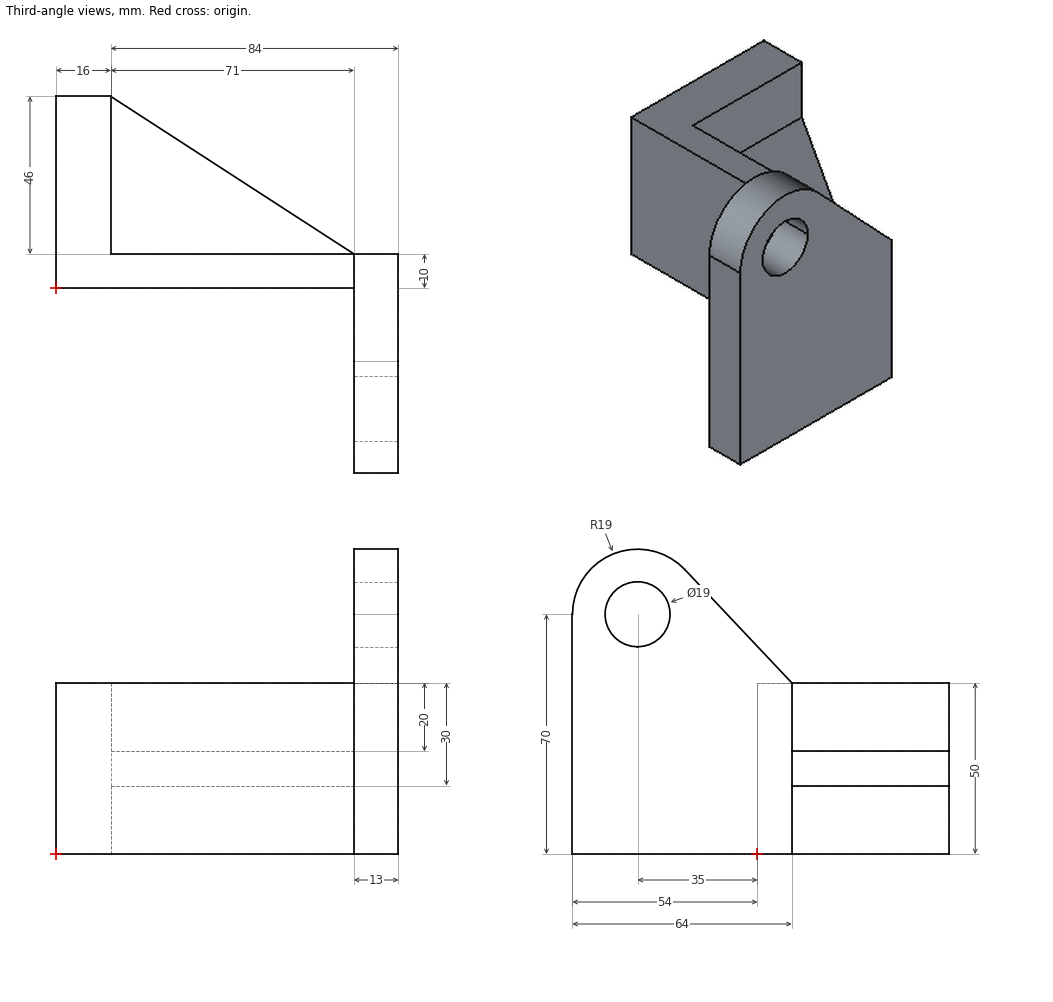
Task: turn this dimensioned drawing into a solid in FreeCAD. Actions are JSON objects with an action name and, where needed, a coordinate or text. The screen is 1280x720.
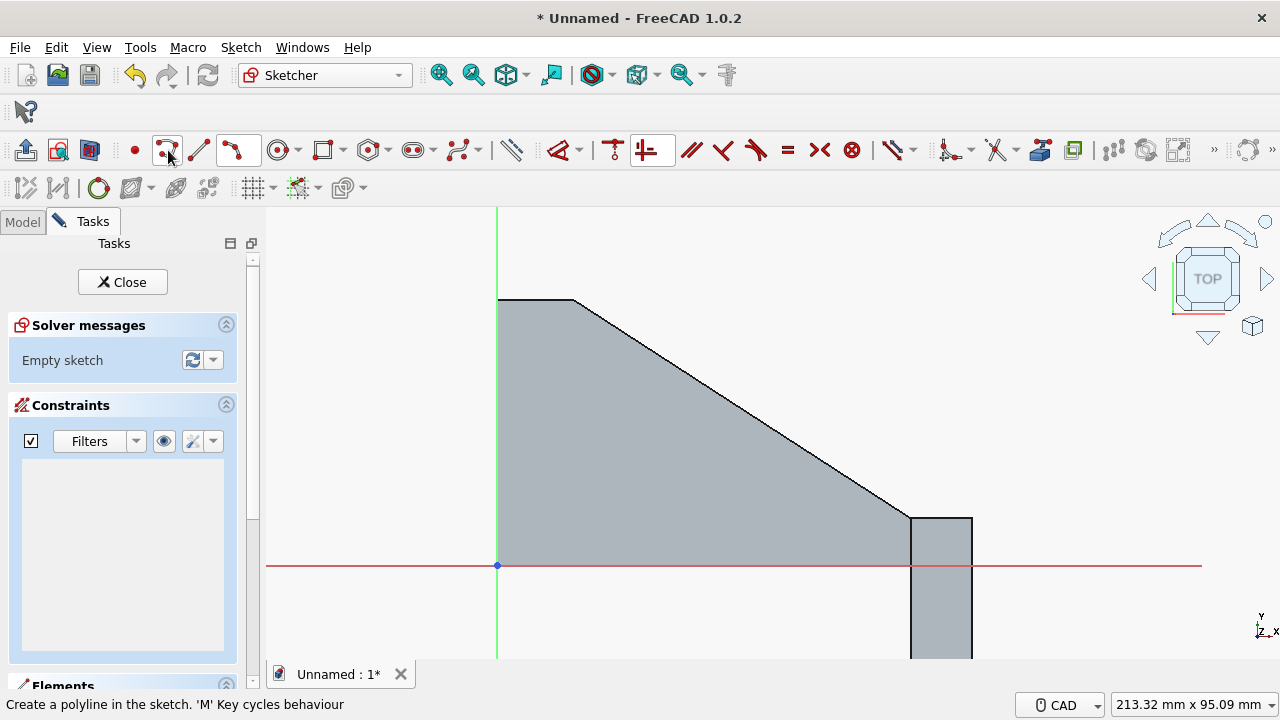
{"action": "left_click", "coordinate": [573, 518]}
{"action": "left_click", "coordinate": [911, 518]}
{"action": "left_click", "coordinate": [573, 300]}
{"action": "left_click", "coordinate": [573, 519]}
{"action": "key", "text": "Escape"}
{"action": "key", "text": "Escape"}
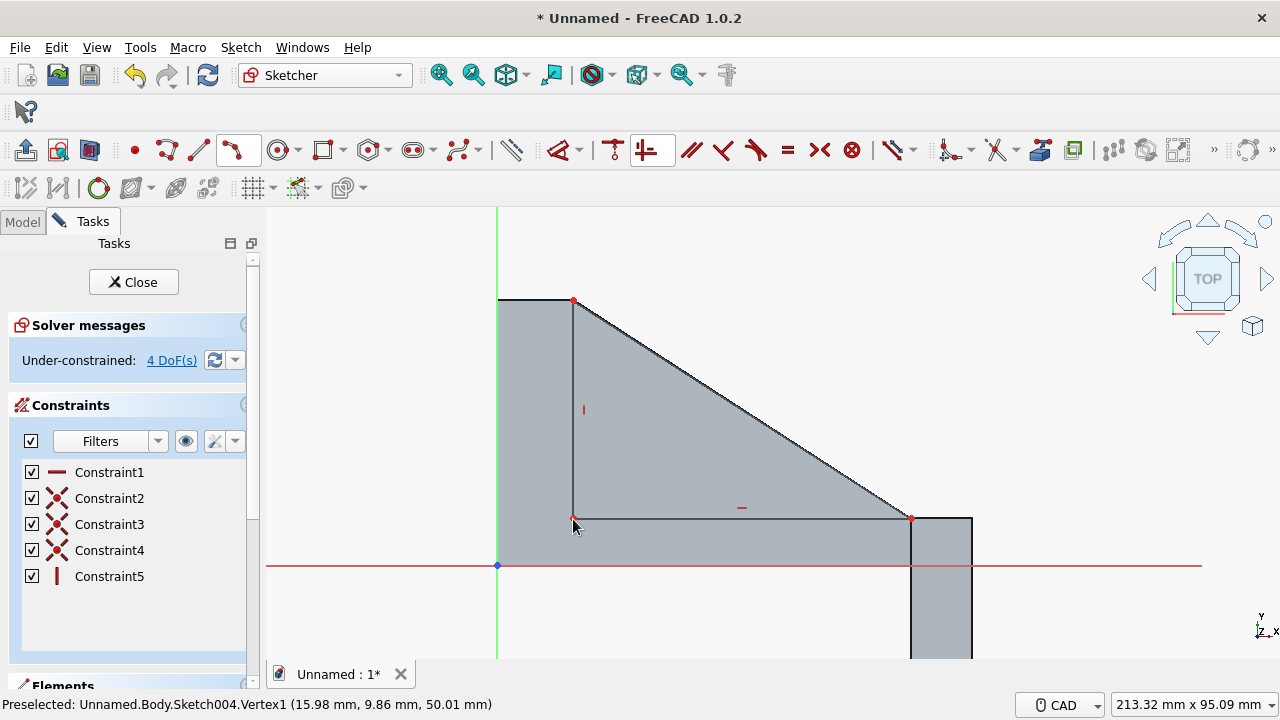
{"action": "key", "text": "d"}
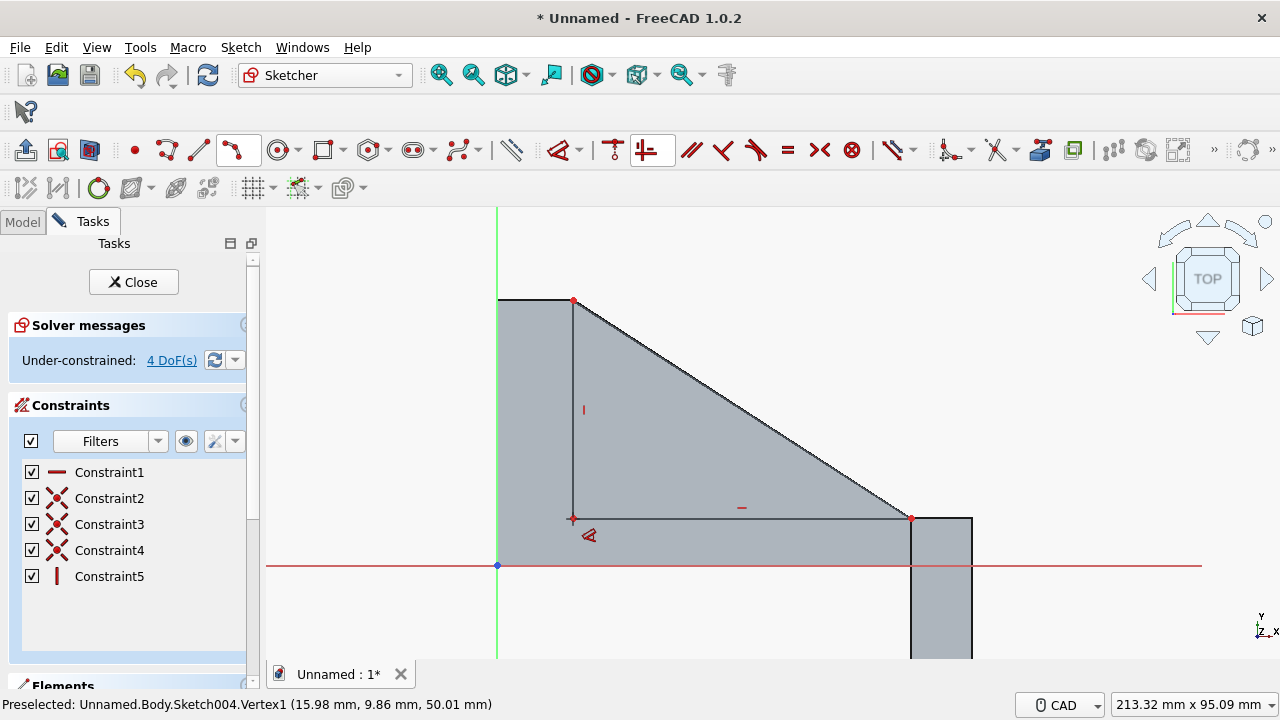
{"action": "left_click", "coordinate": [674, 519]}
{"action": "left_click", "coordinate": [742, 485]}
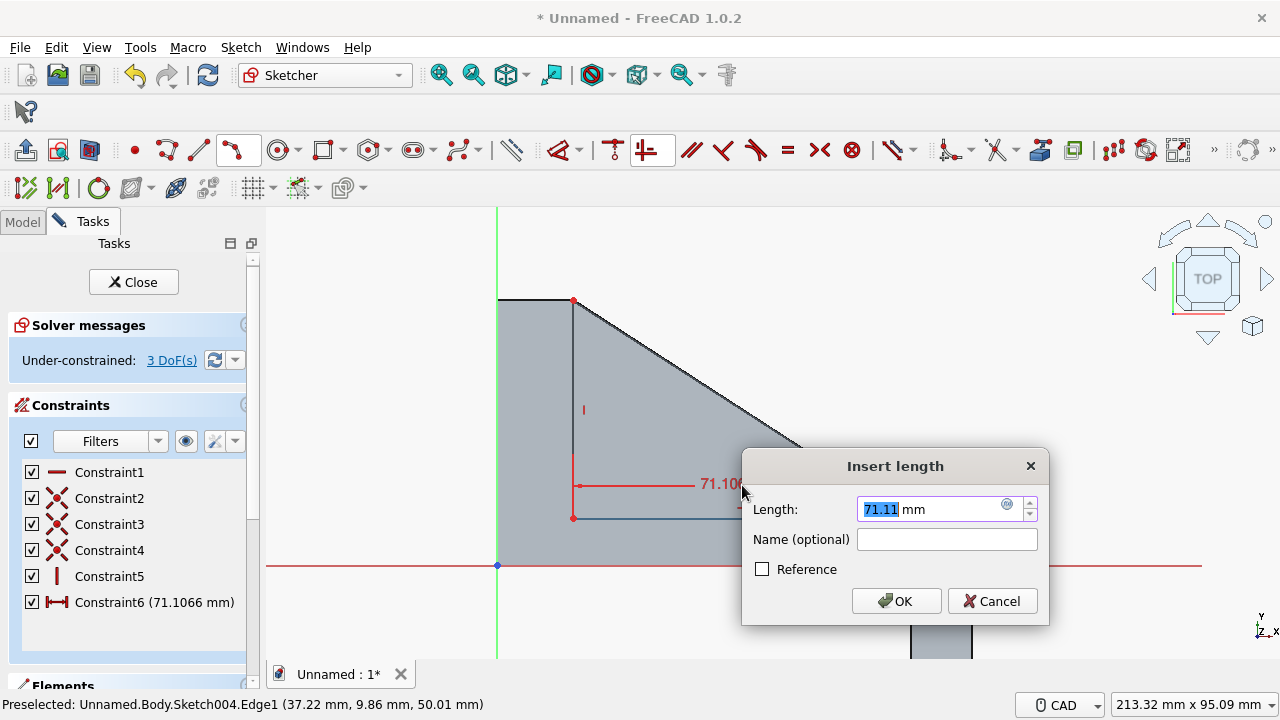
{"action": "type", "text": "71"}
{"action": "key", "text": "Return"}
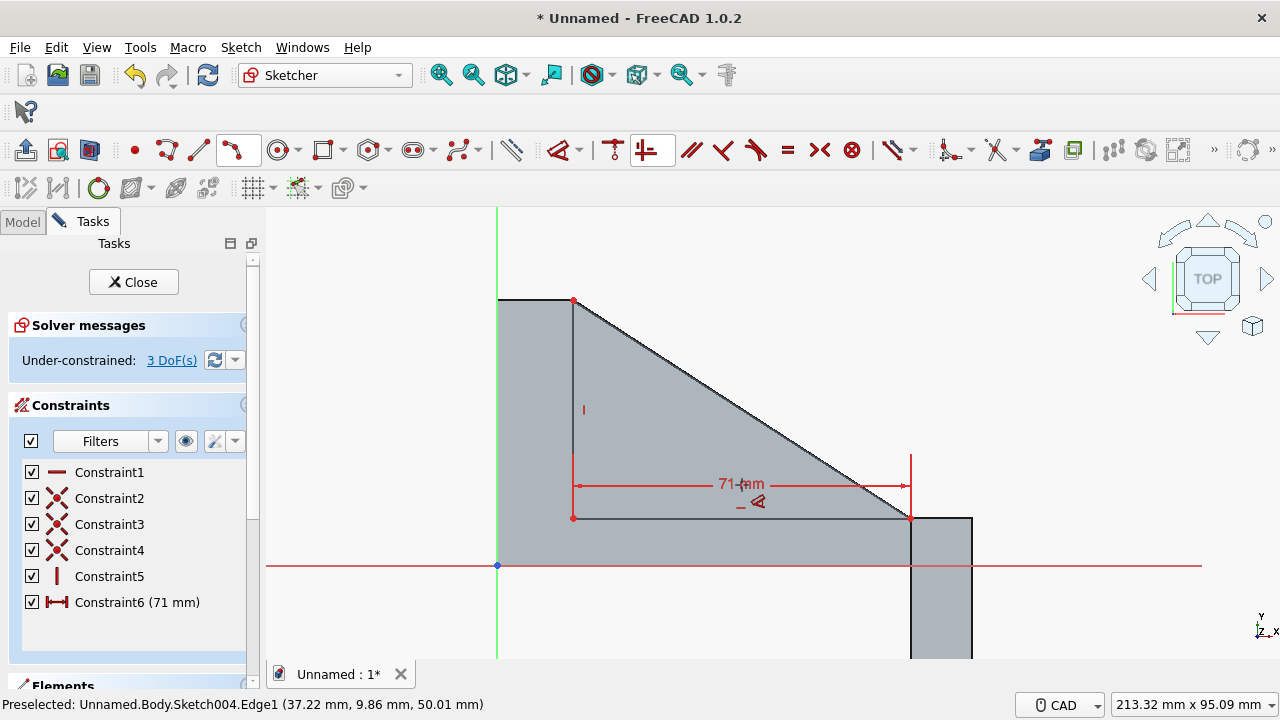
{"action": "left_click", "coordinate": [573, 366]}
{"action": "left_click", "coordinate": [539, 410]}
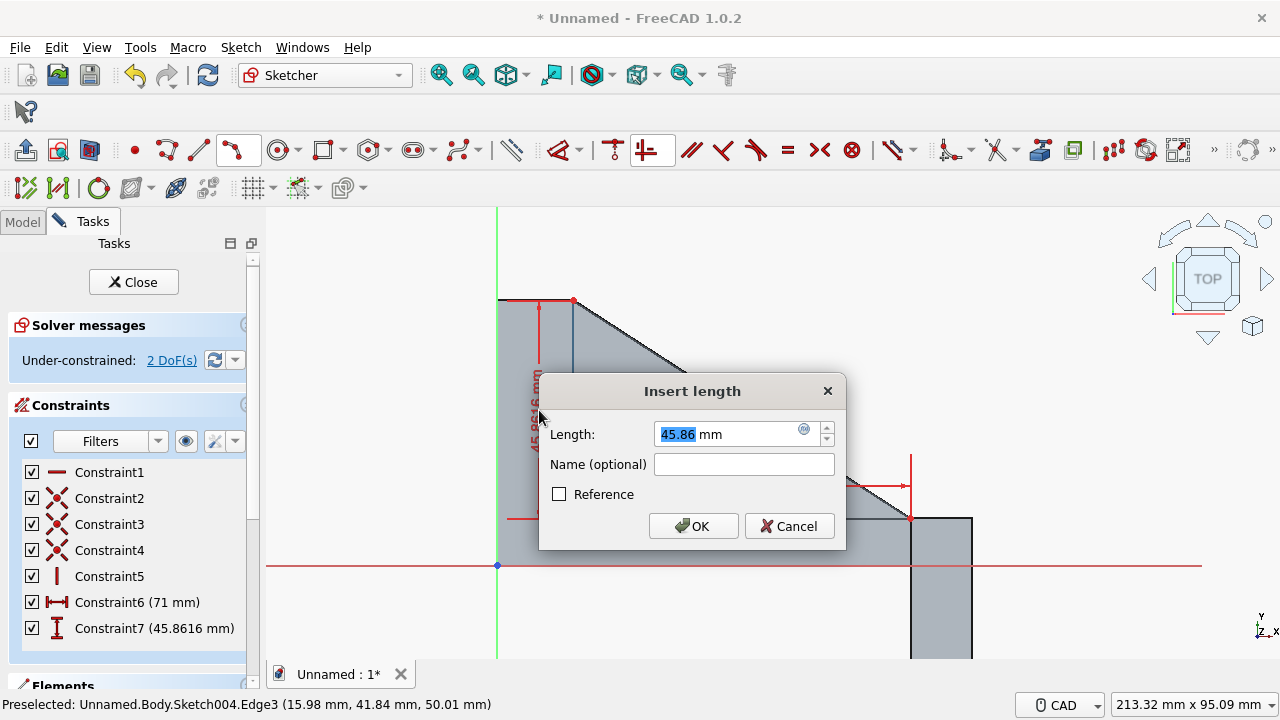
{"action": "type", "text": "46"}
{"action": "key", "text": "Return"}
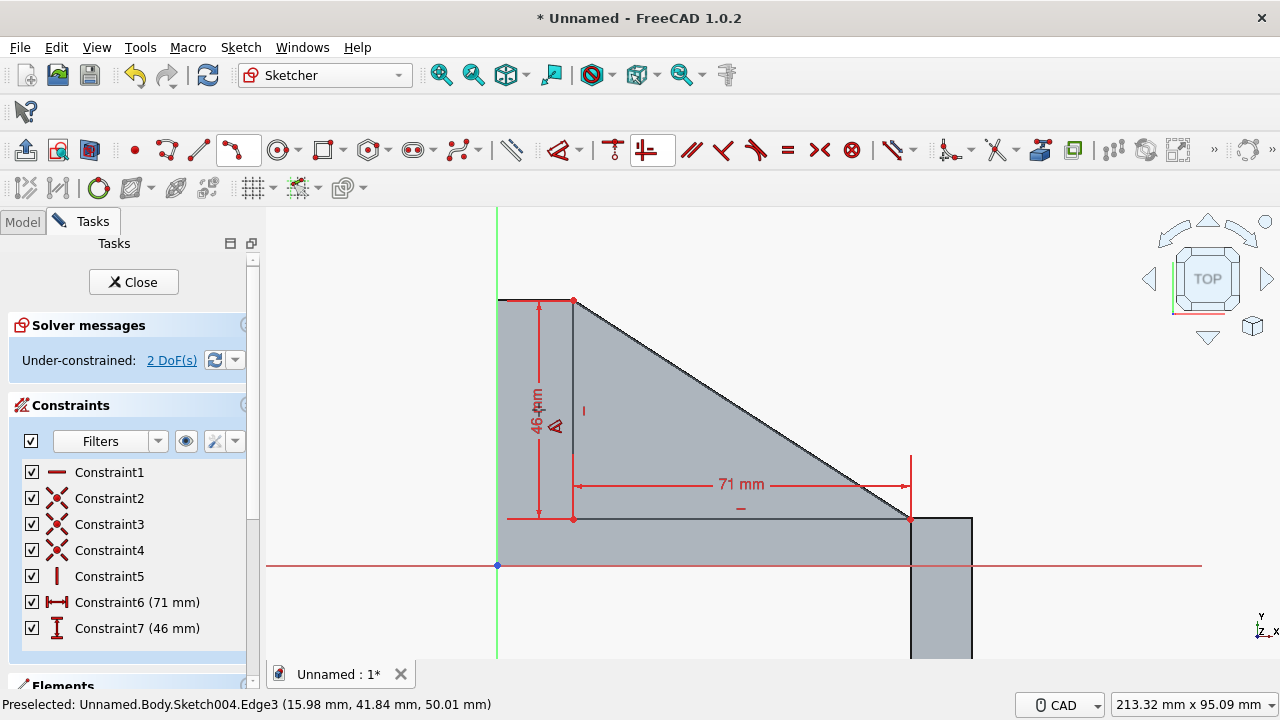
{"action": "left_click", "coordinate": [573, 519]}
{"action": "left_click", "coordinate": [535, 600]}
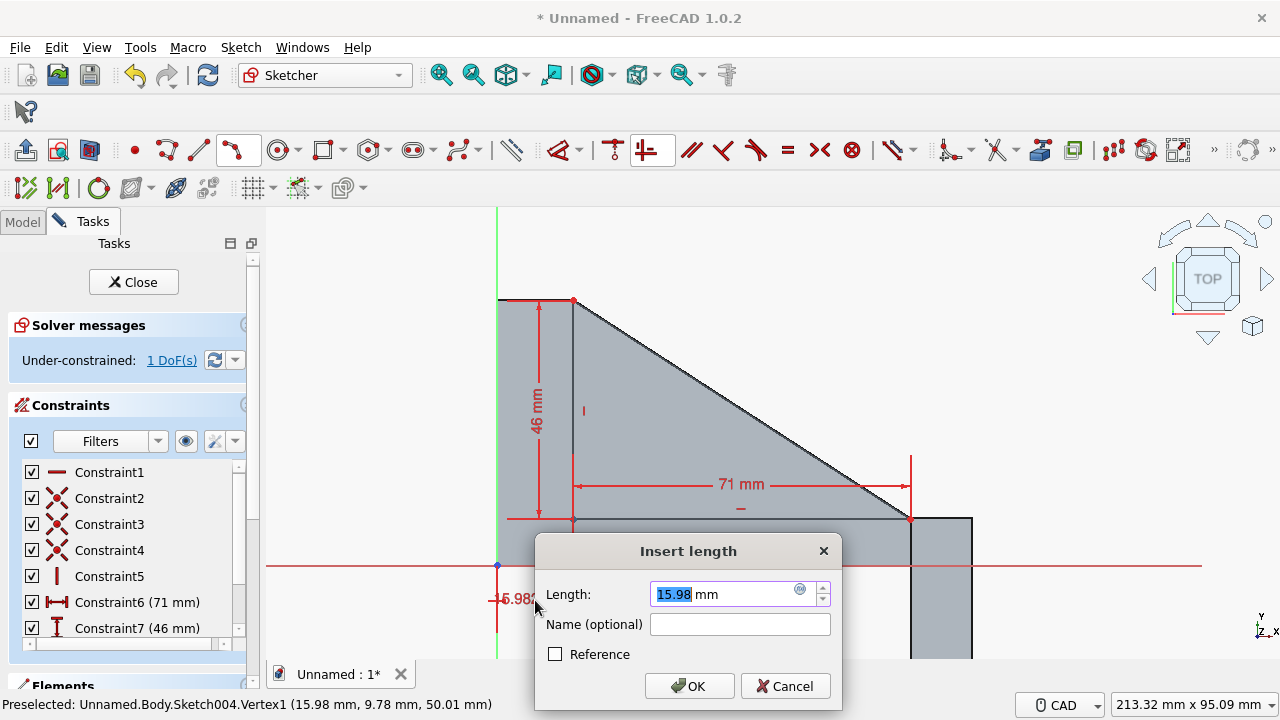
{"action": "type", "text": "16"}
{"action": "key", "text": "Return"}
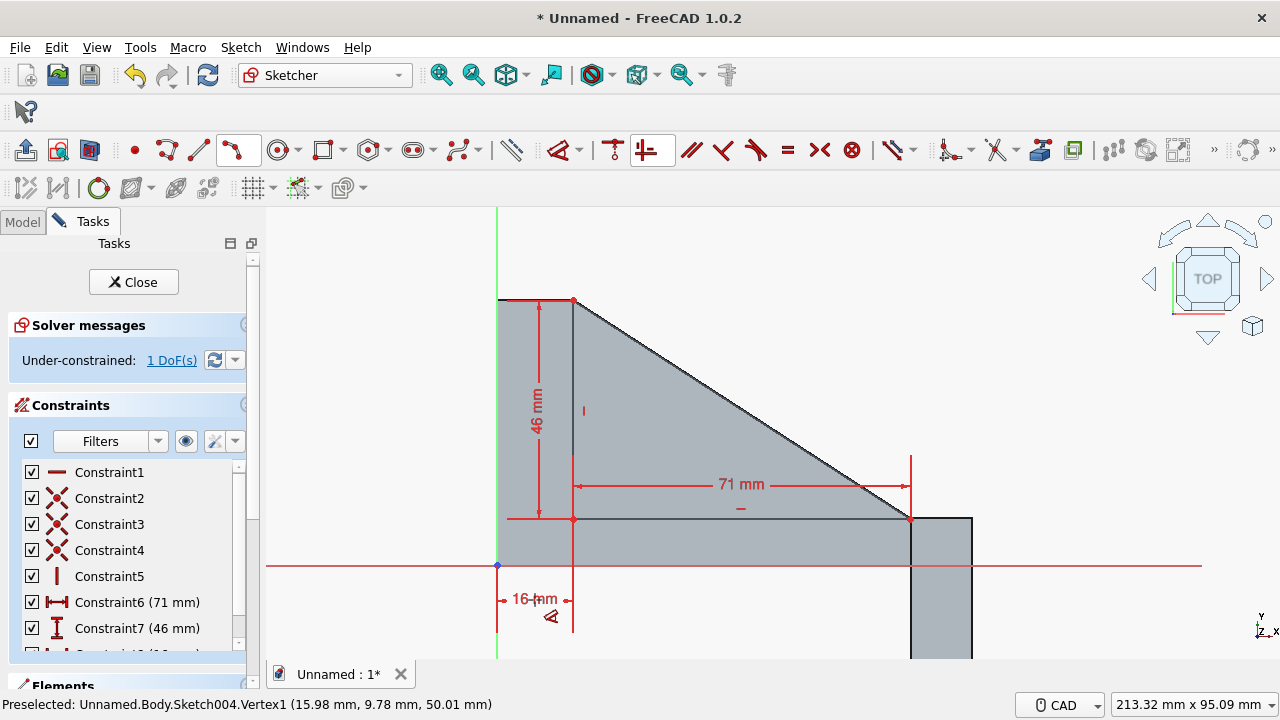
{"action": "left_click", "coordinate": [573, 519]}
{"action": "left_click", "coordinate": [463, 543]}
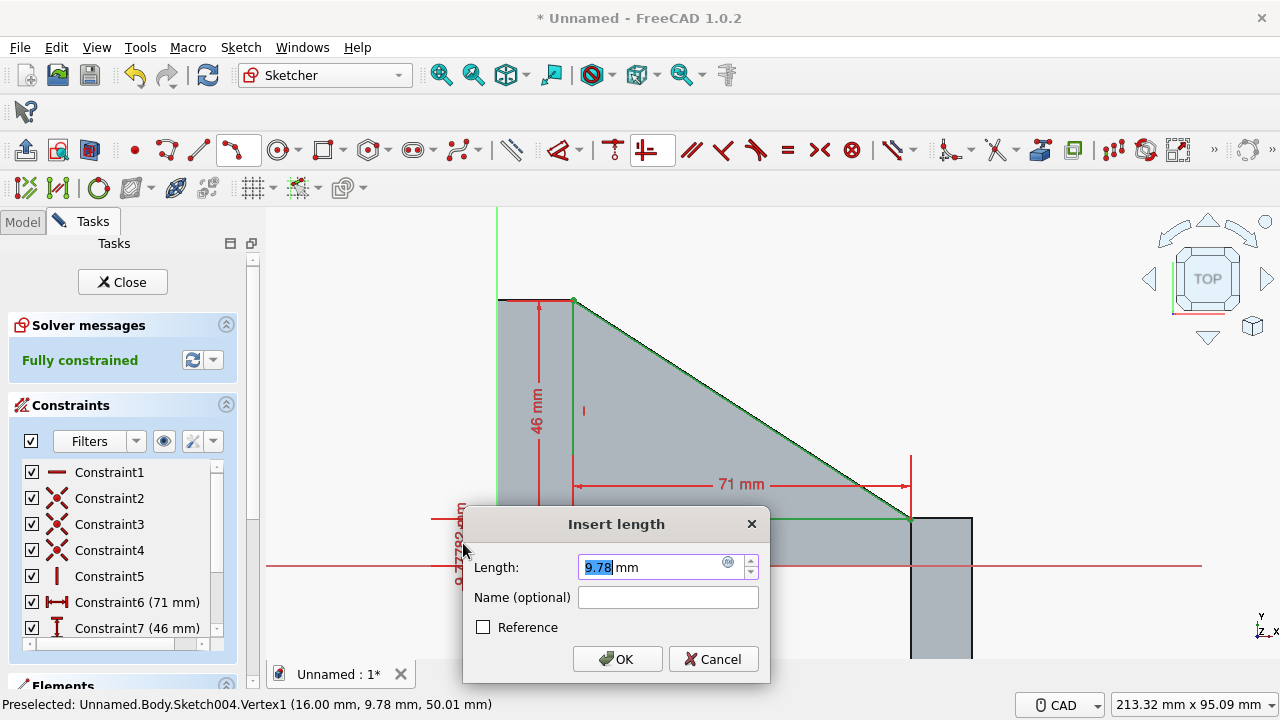
{"action": "type", "text": "10"}
{"action": "key", "text": "Return"}
{"action": "key", "text": "Escape"}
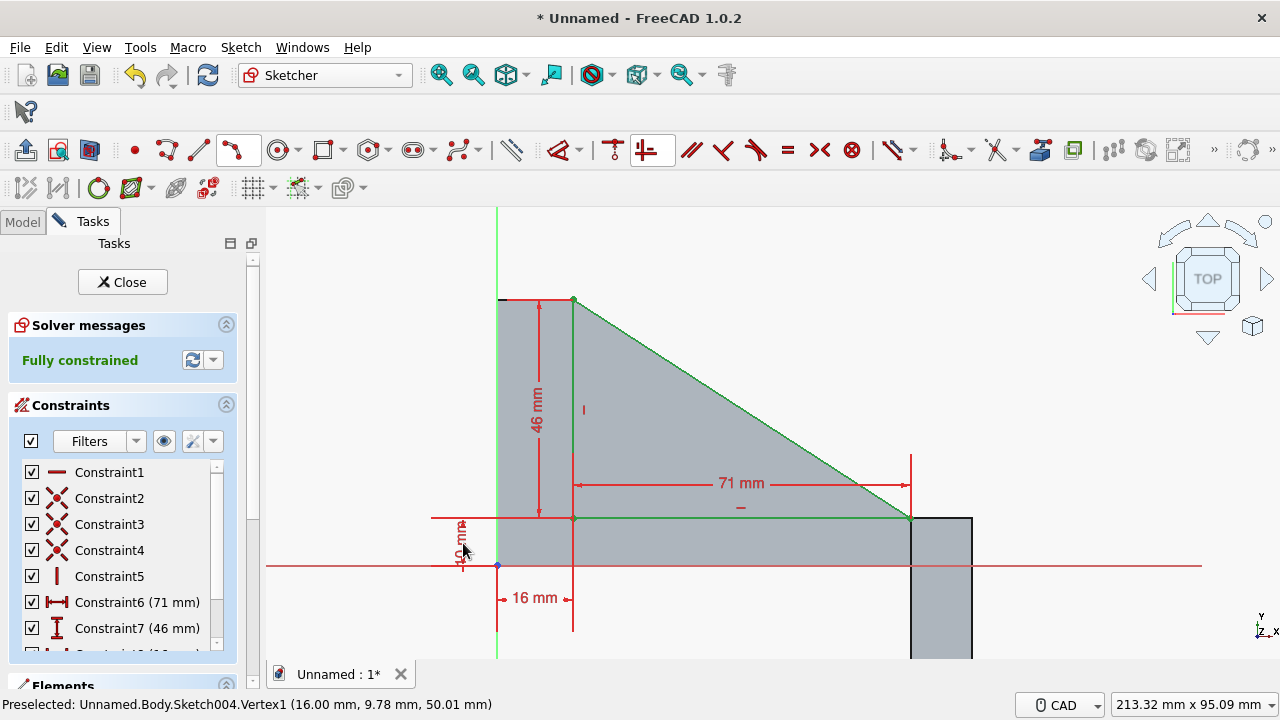
{"action": "left_click", "coordinate": [123, 282]}